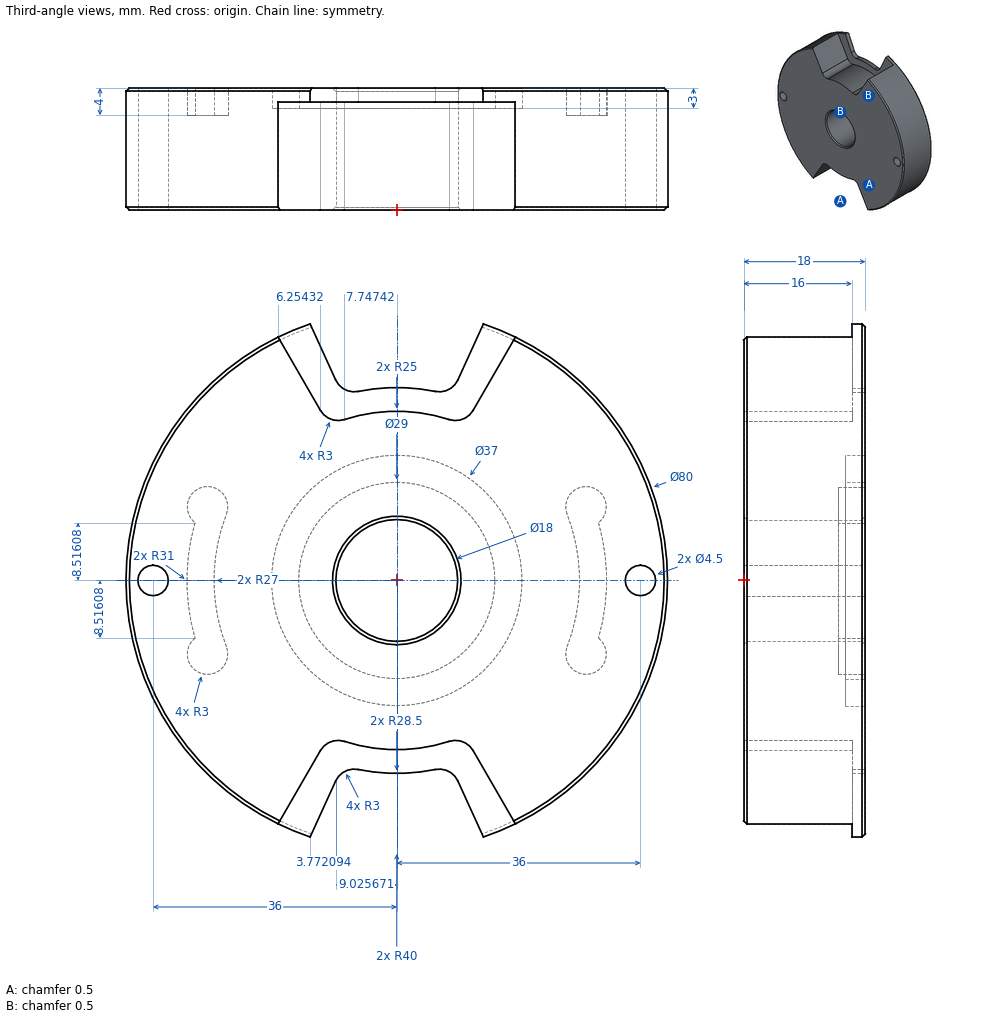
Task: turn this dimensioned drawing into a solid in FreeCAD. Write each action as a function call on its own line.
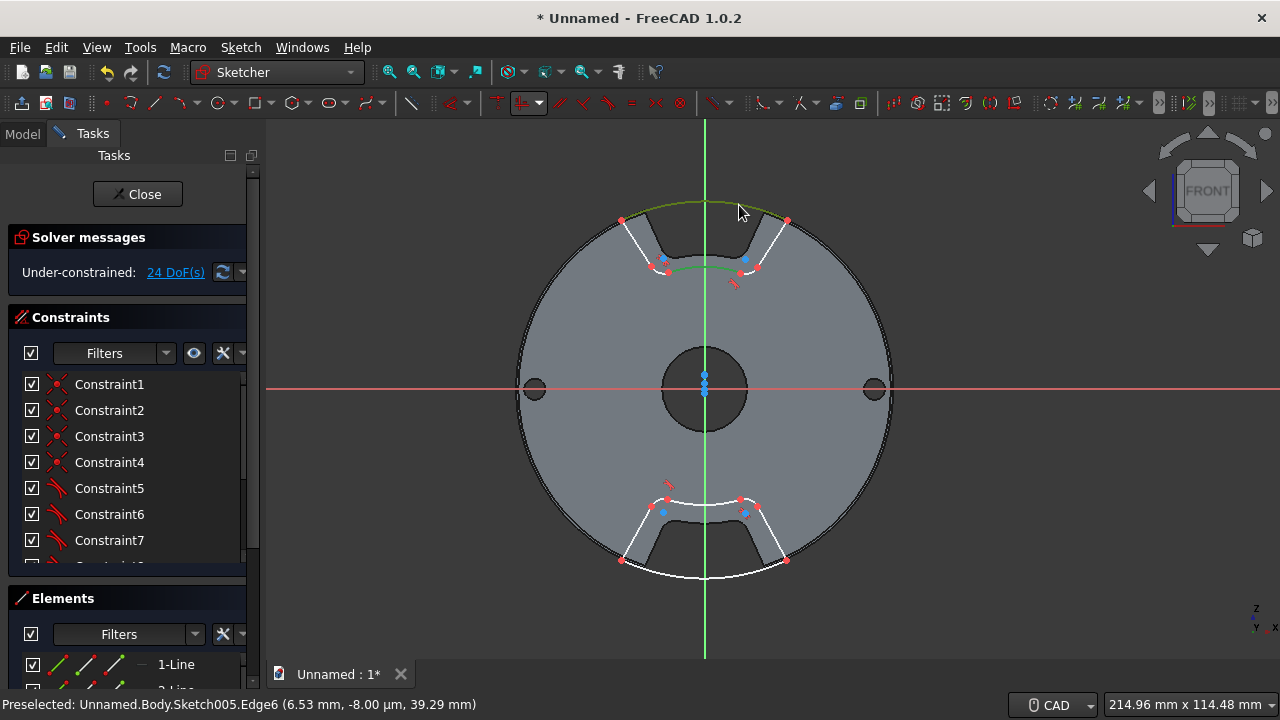
click(498, 104)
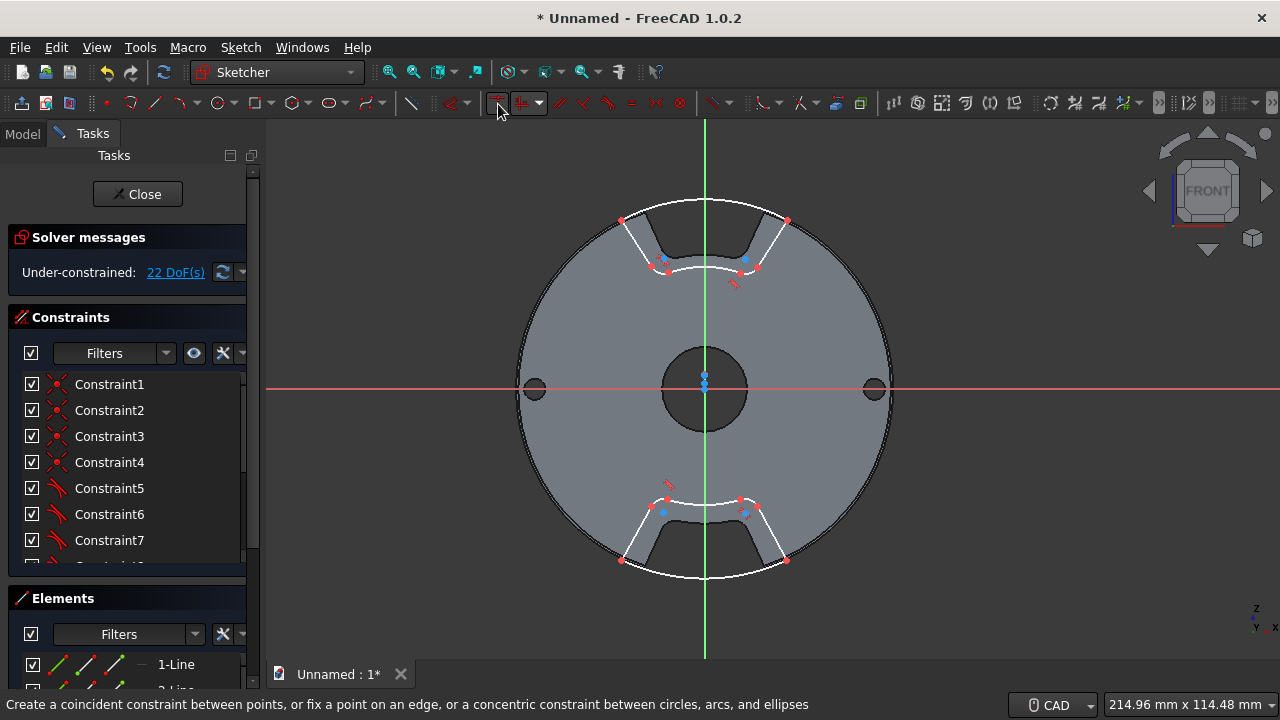
click(719, 268)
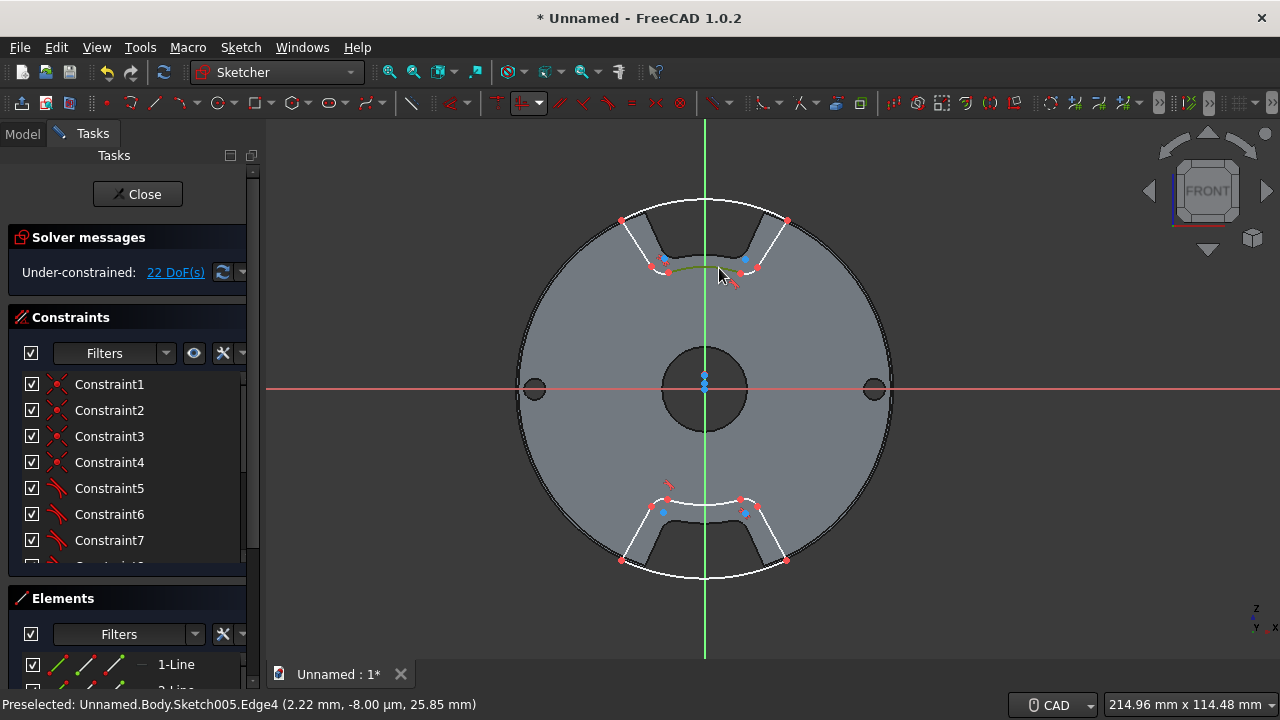
click(689, 504)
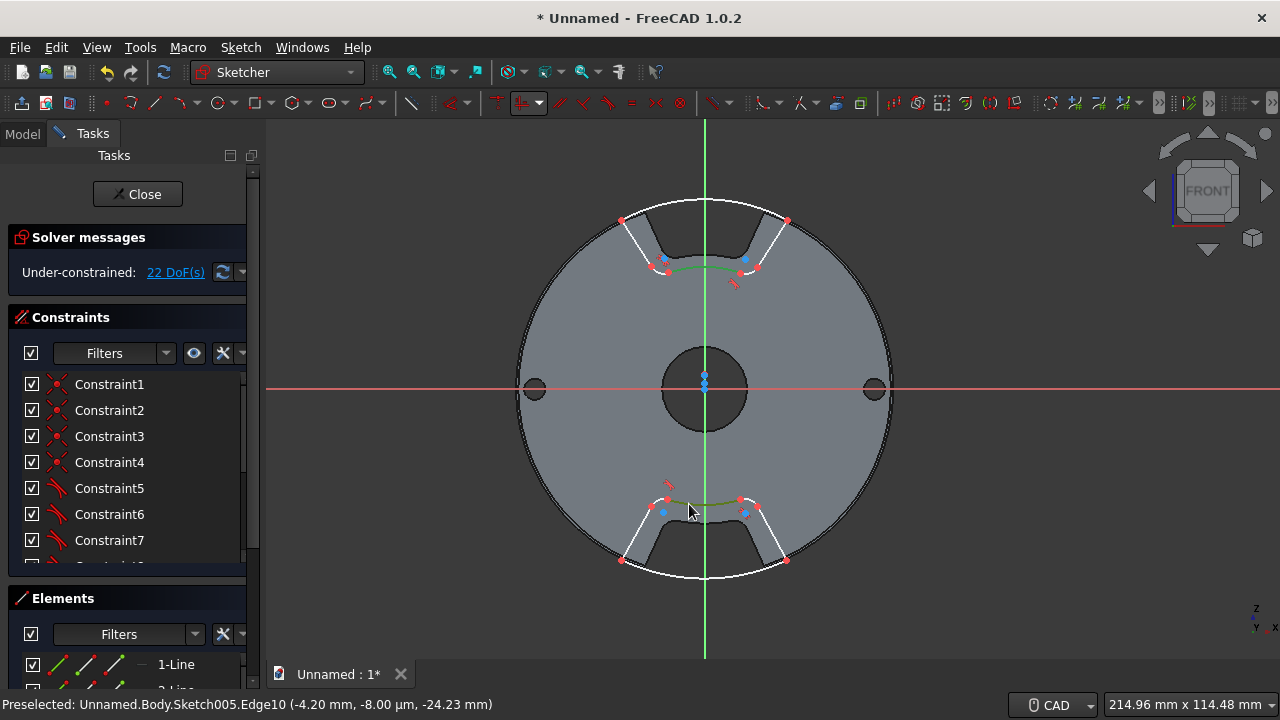
click(498, 104)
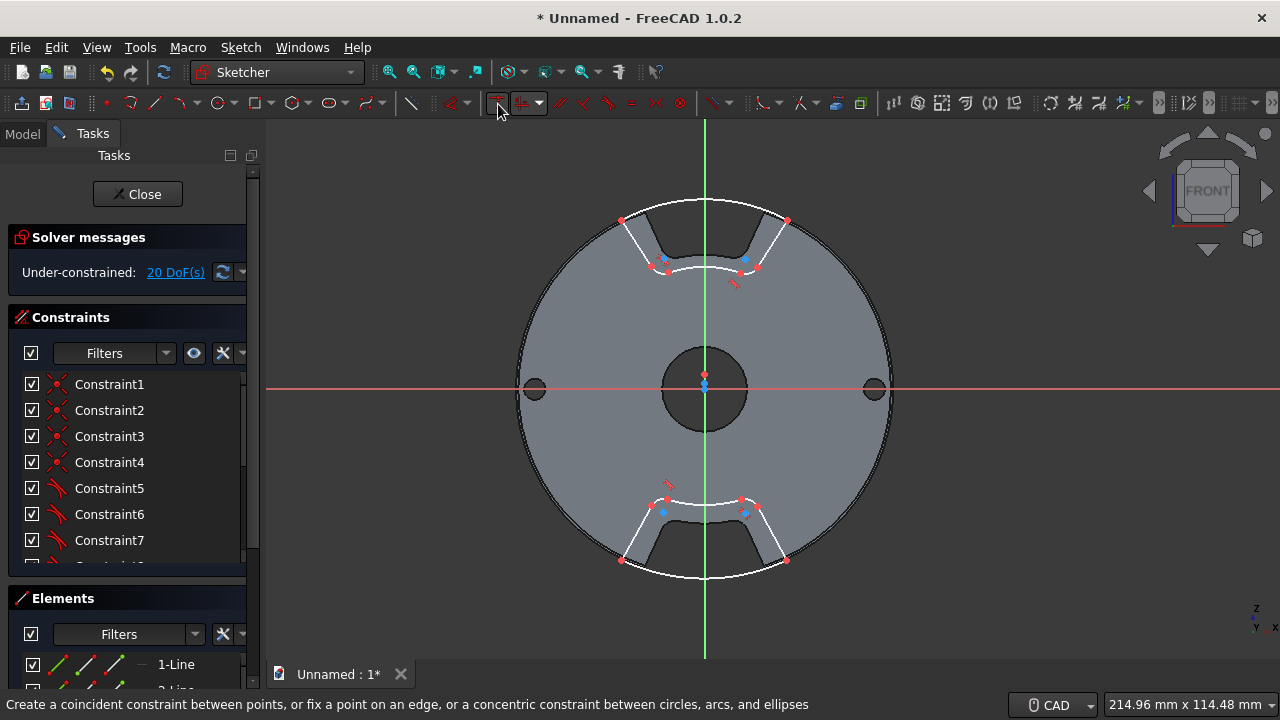
click(719, 268)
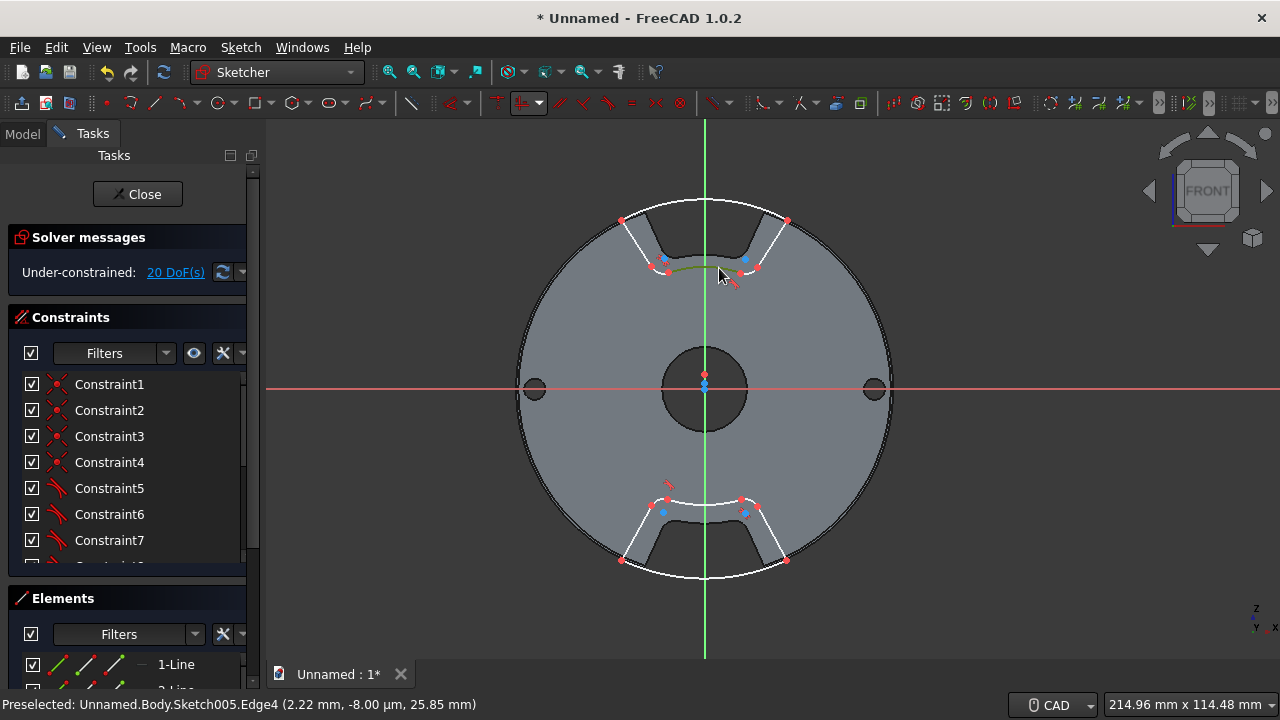
click(670, 576)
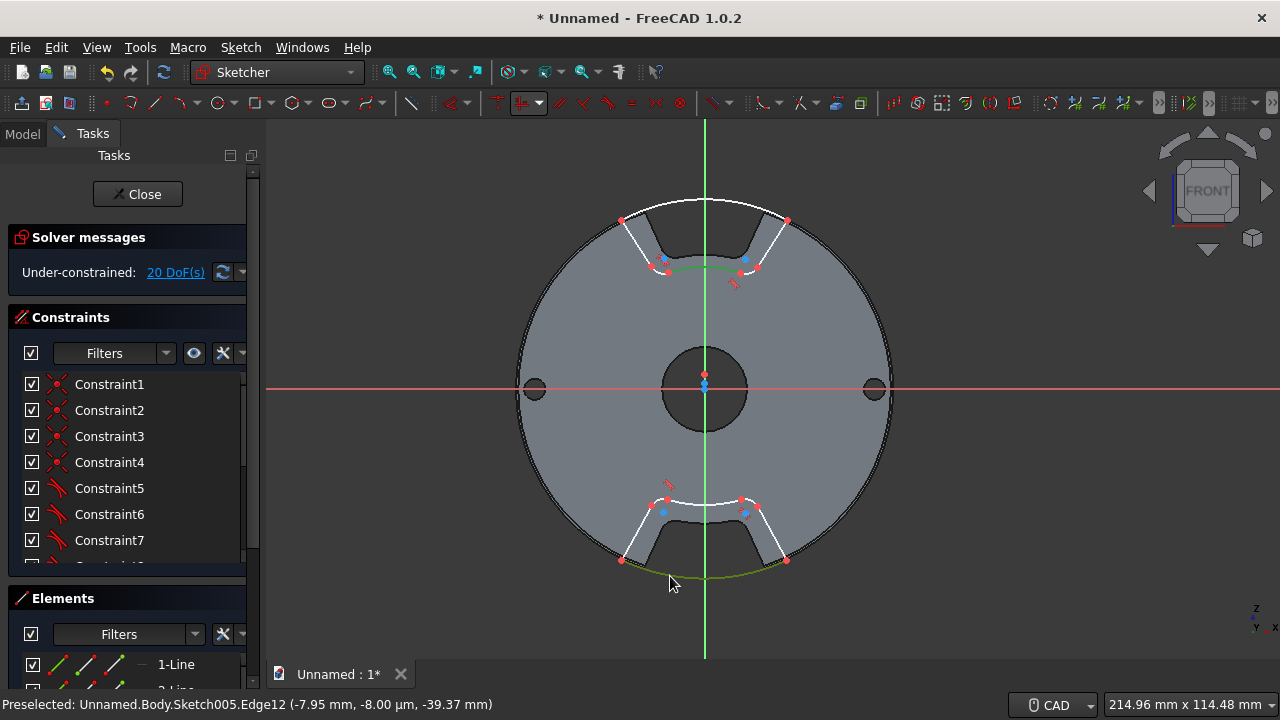
click(498, 104)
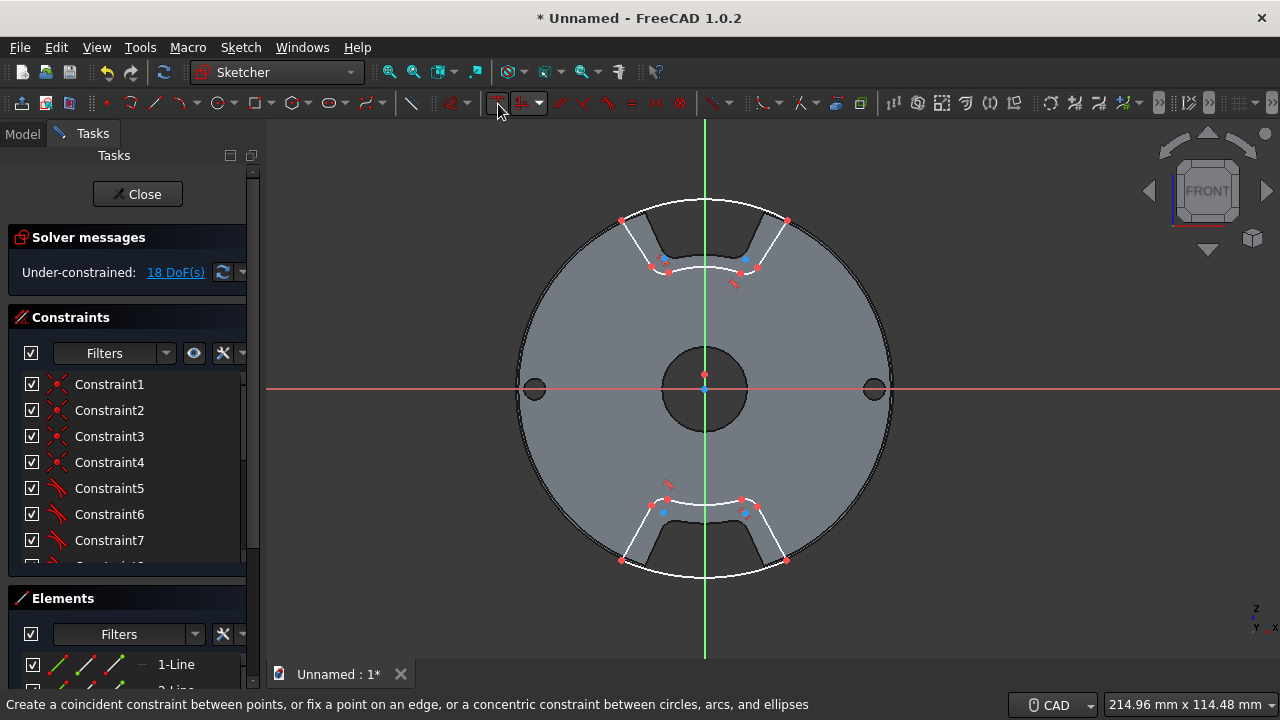
scroll(705, 382, up, 6)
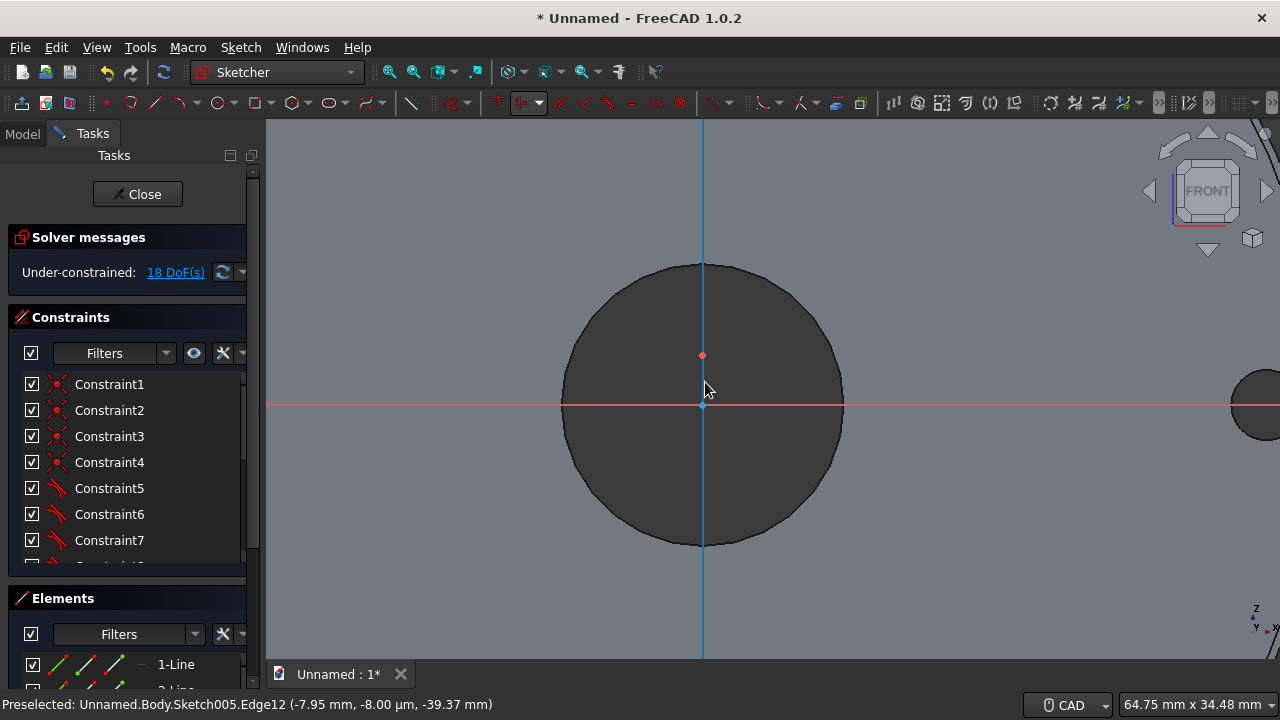
drag(693, 346, 713, 415)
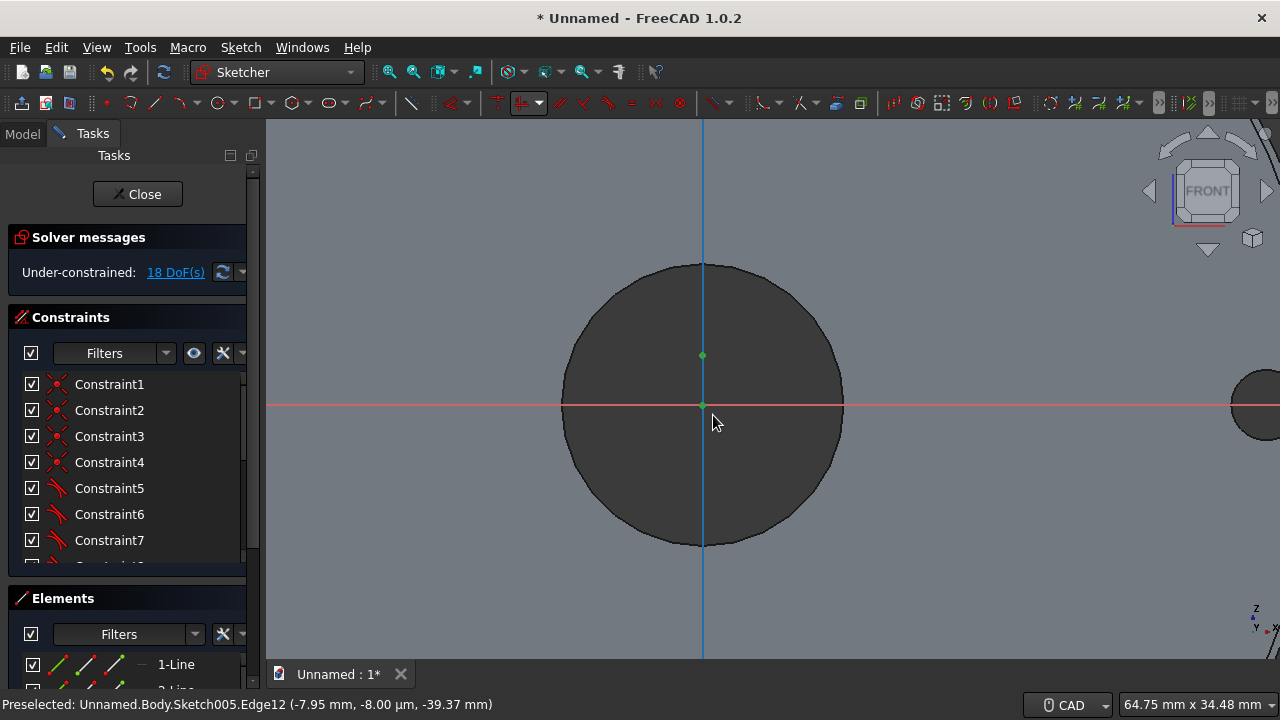
click(498, 104)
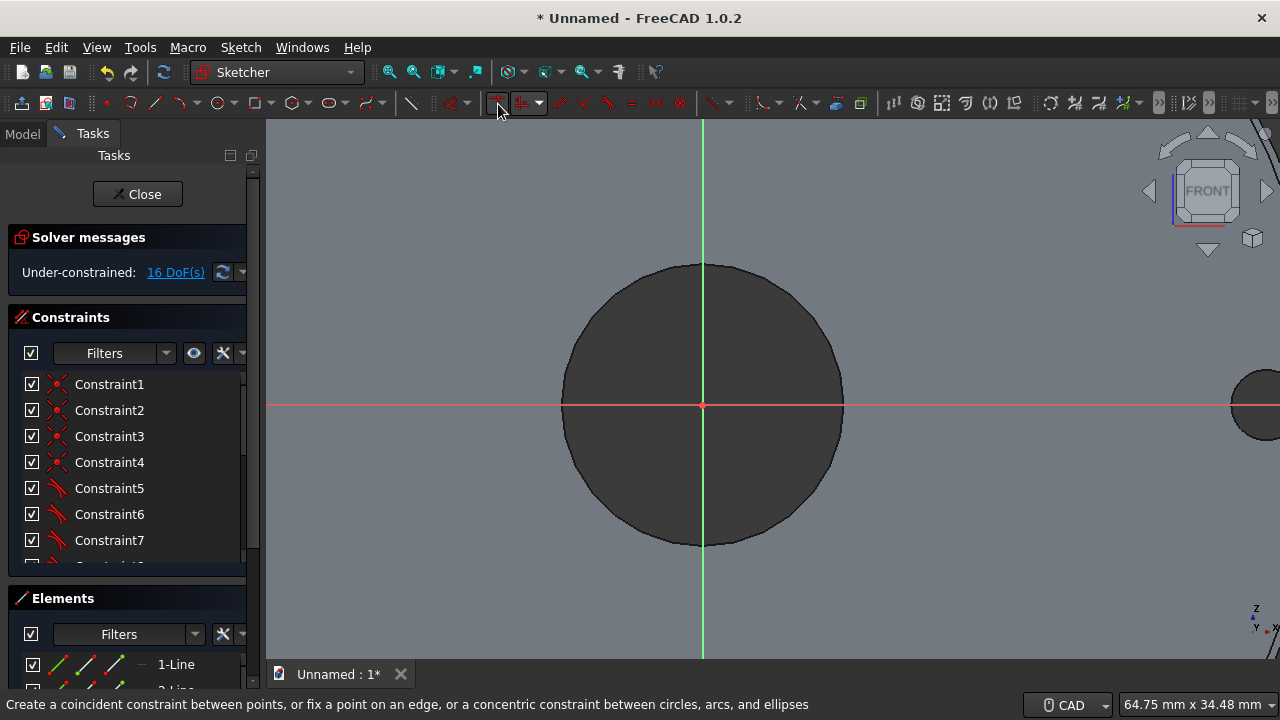
scroll(705, 382, down, 6)